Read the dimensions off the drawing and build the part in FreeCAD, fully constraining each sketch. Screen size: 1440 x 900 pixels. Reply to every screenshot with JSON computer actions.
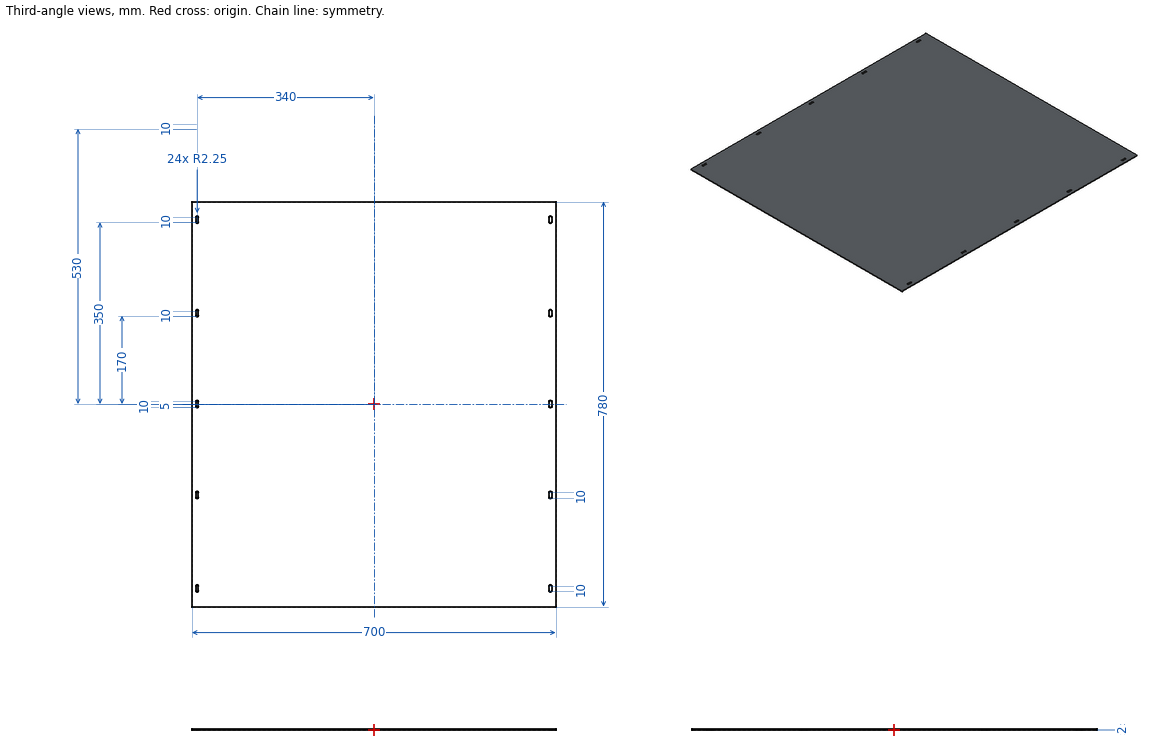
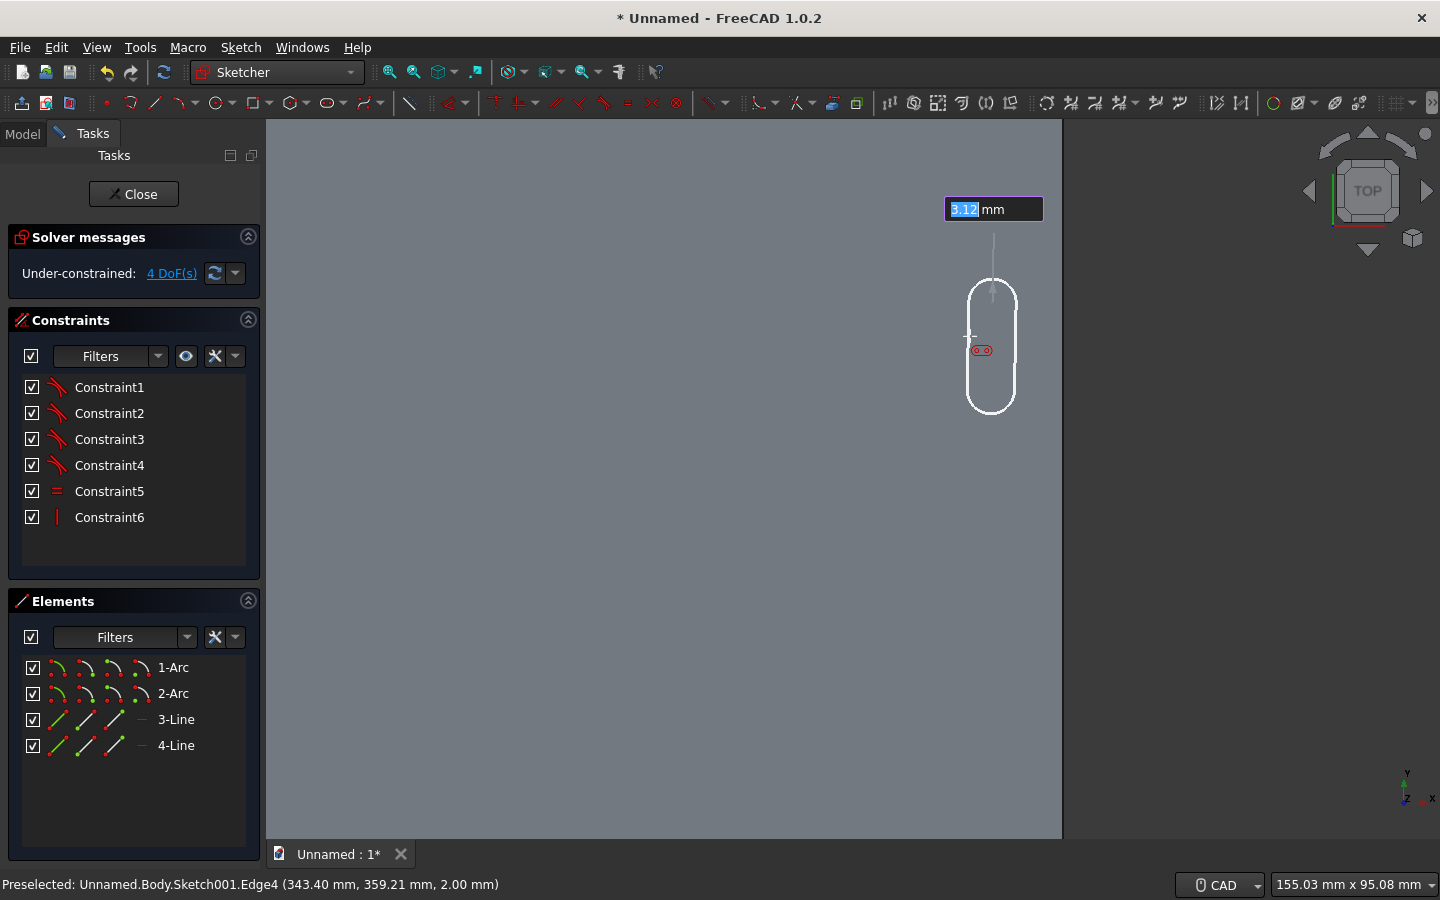
{"action": "left_click", "coordinate": [970, 335]}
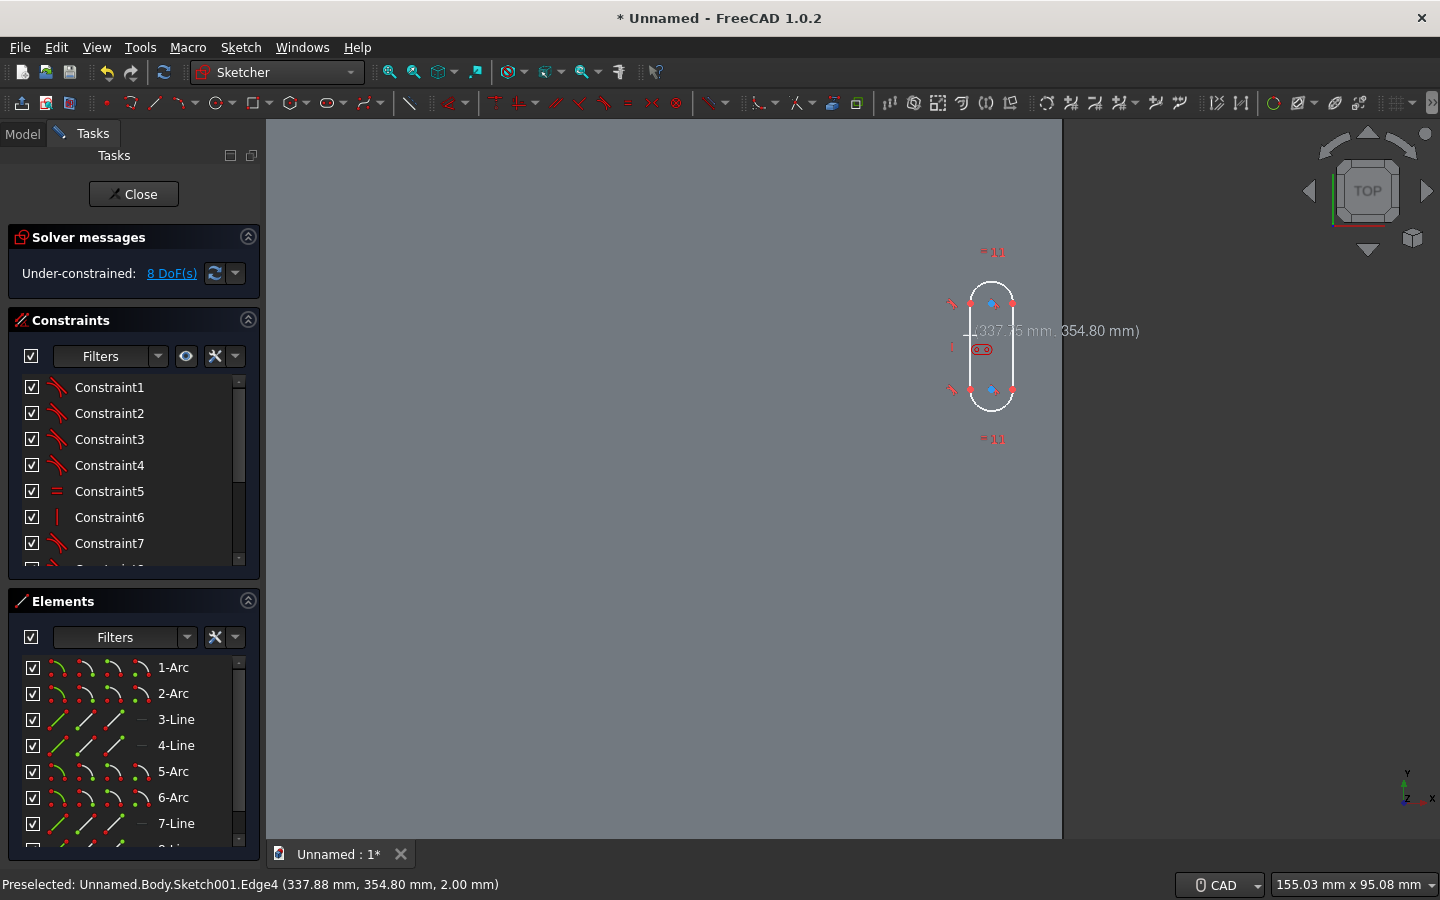
{"action": "scroll", "coordinate": [975, 330], "scroll_direction": "down", "scroll_amount": 13}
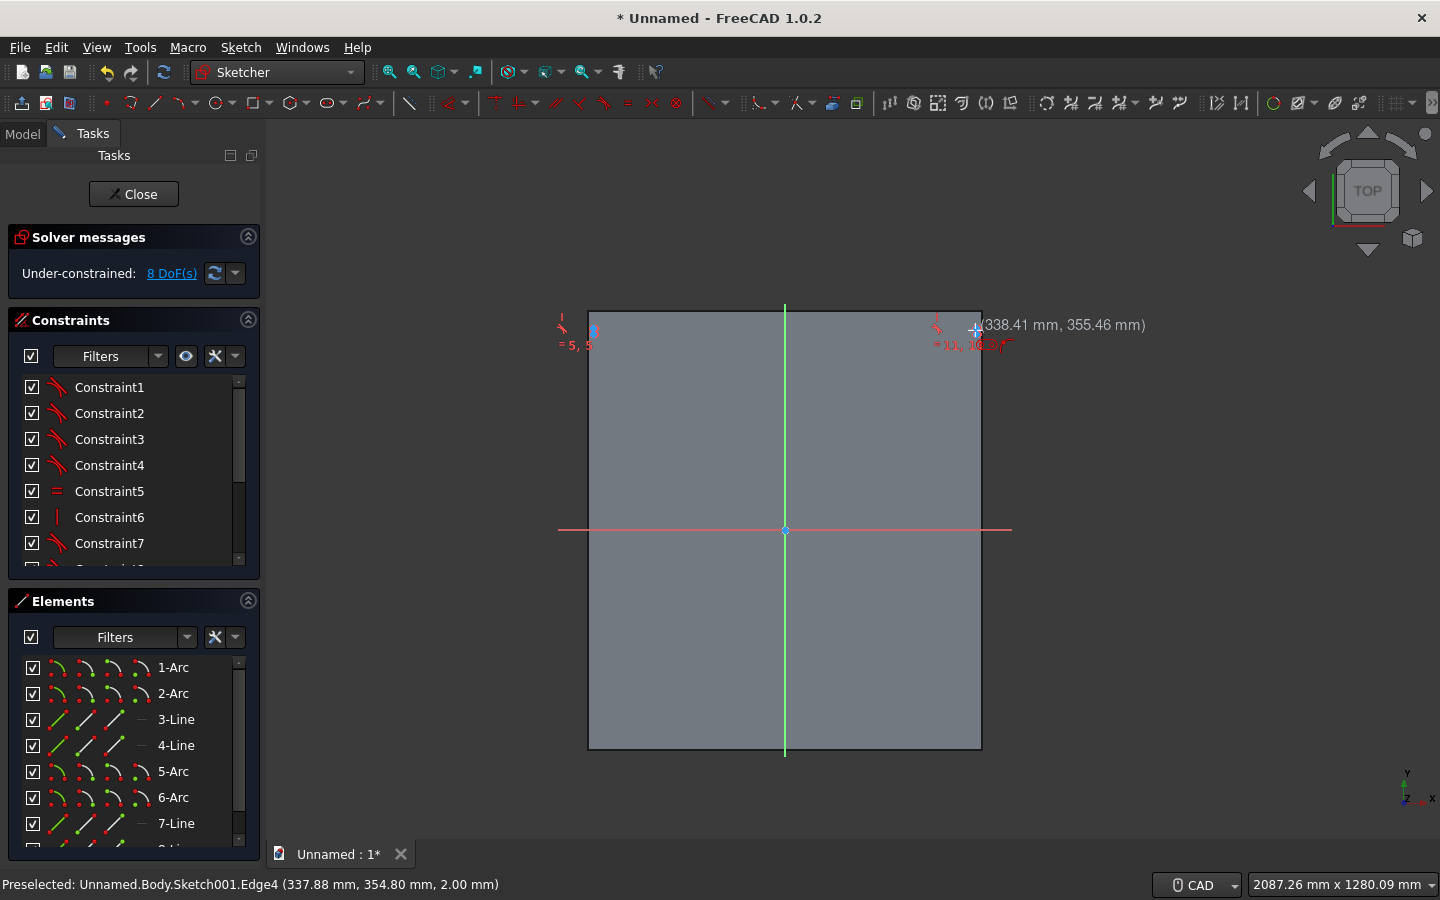
{"action": "scroll", "coordinate": [594, 435], "scroll_direction": "up", "scroll_amount": 15}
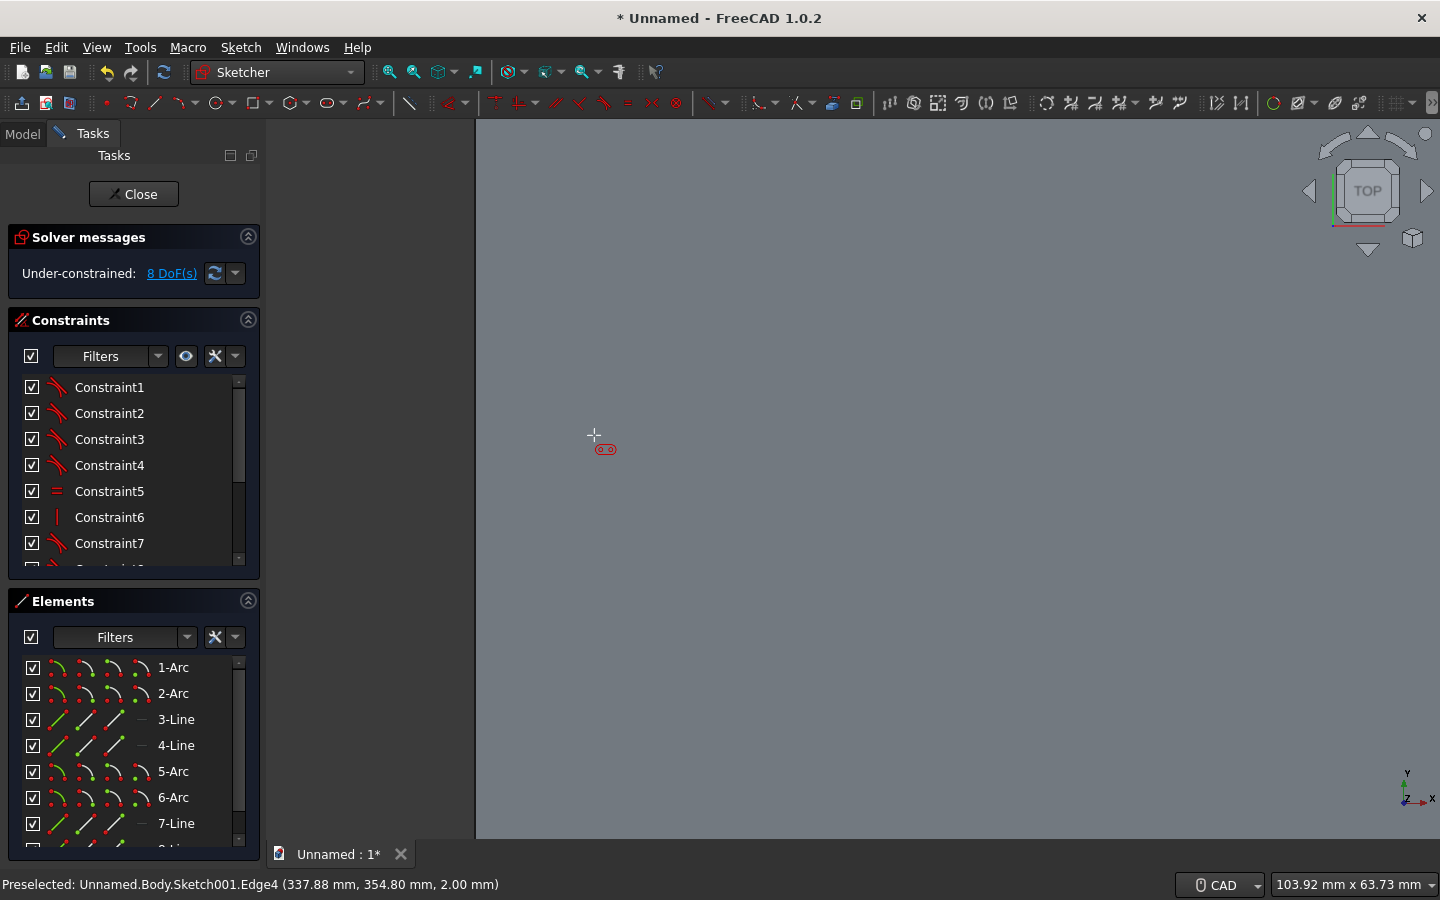
{"action": "scroll", "coordinate": [594, 435], "scroll_direction": "down", "scroll_amount": 15}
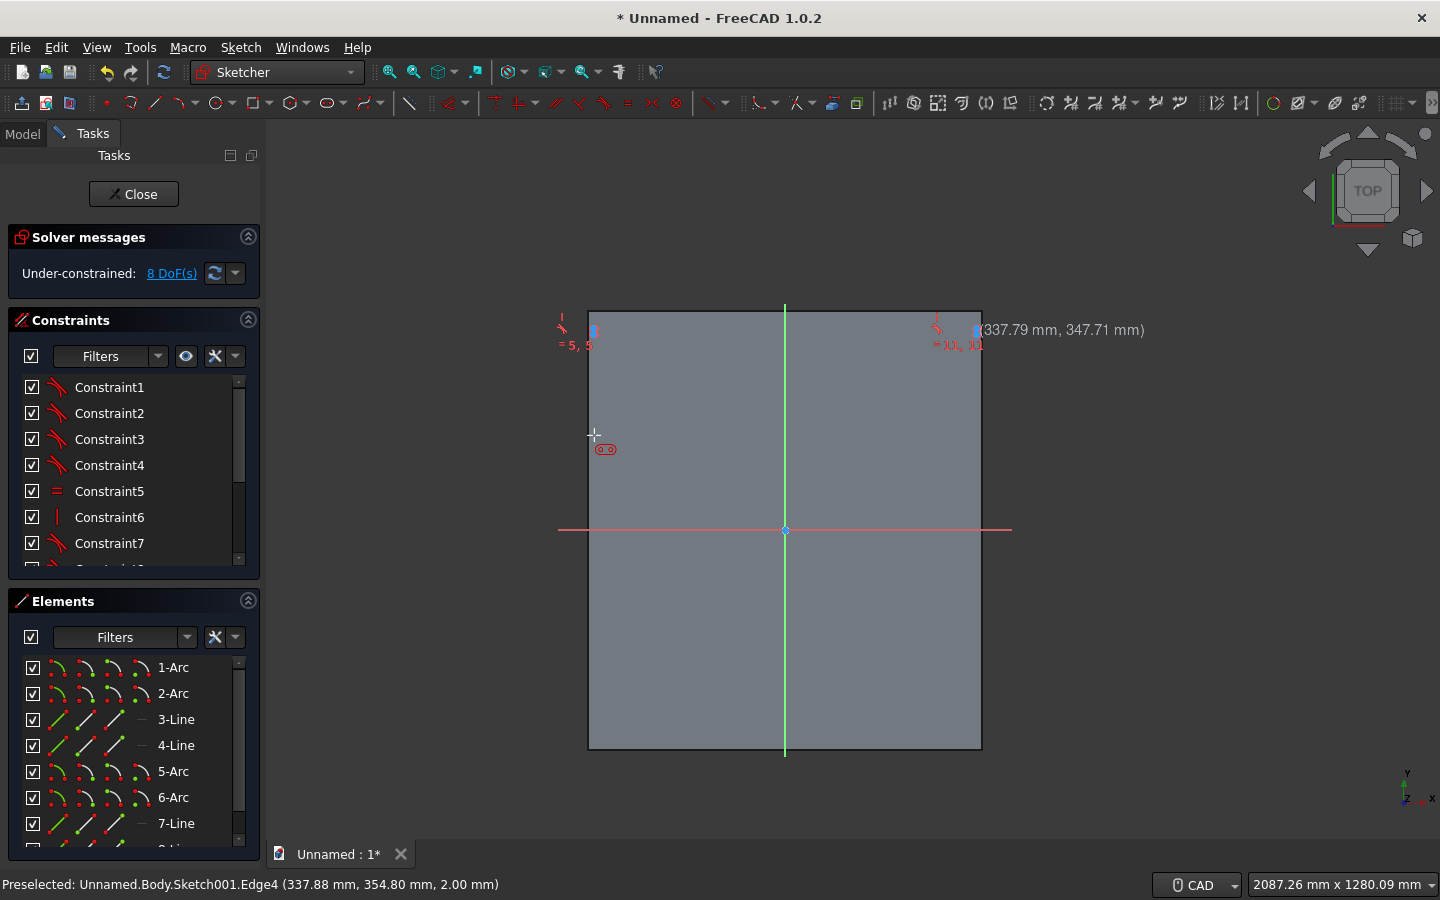
{"action": "left_click", "coordinate": [594, 435]}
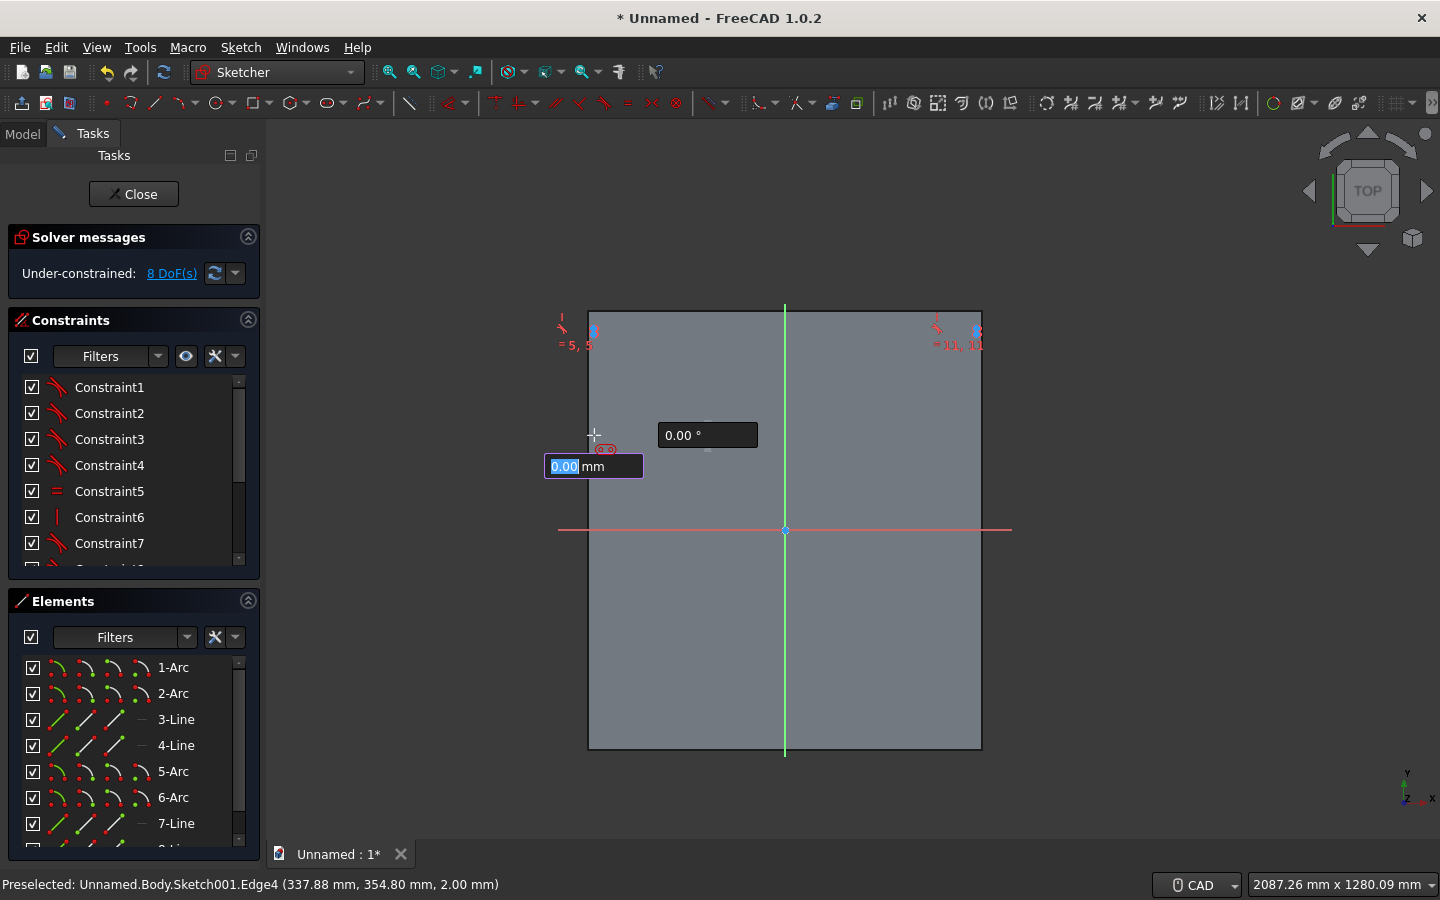
{"action": "scroll", "coordinate": [594, 429], "scroll_direction": "up", "scroll_amount": 6}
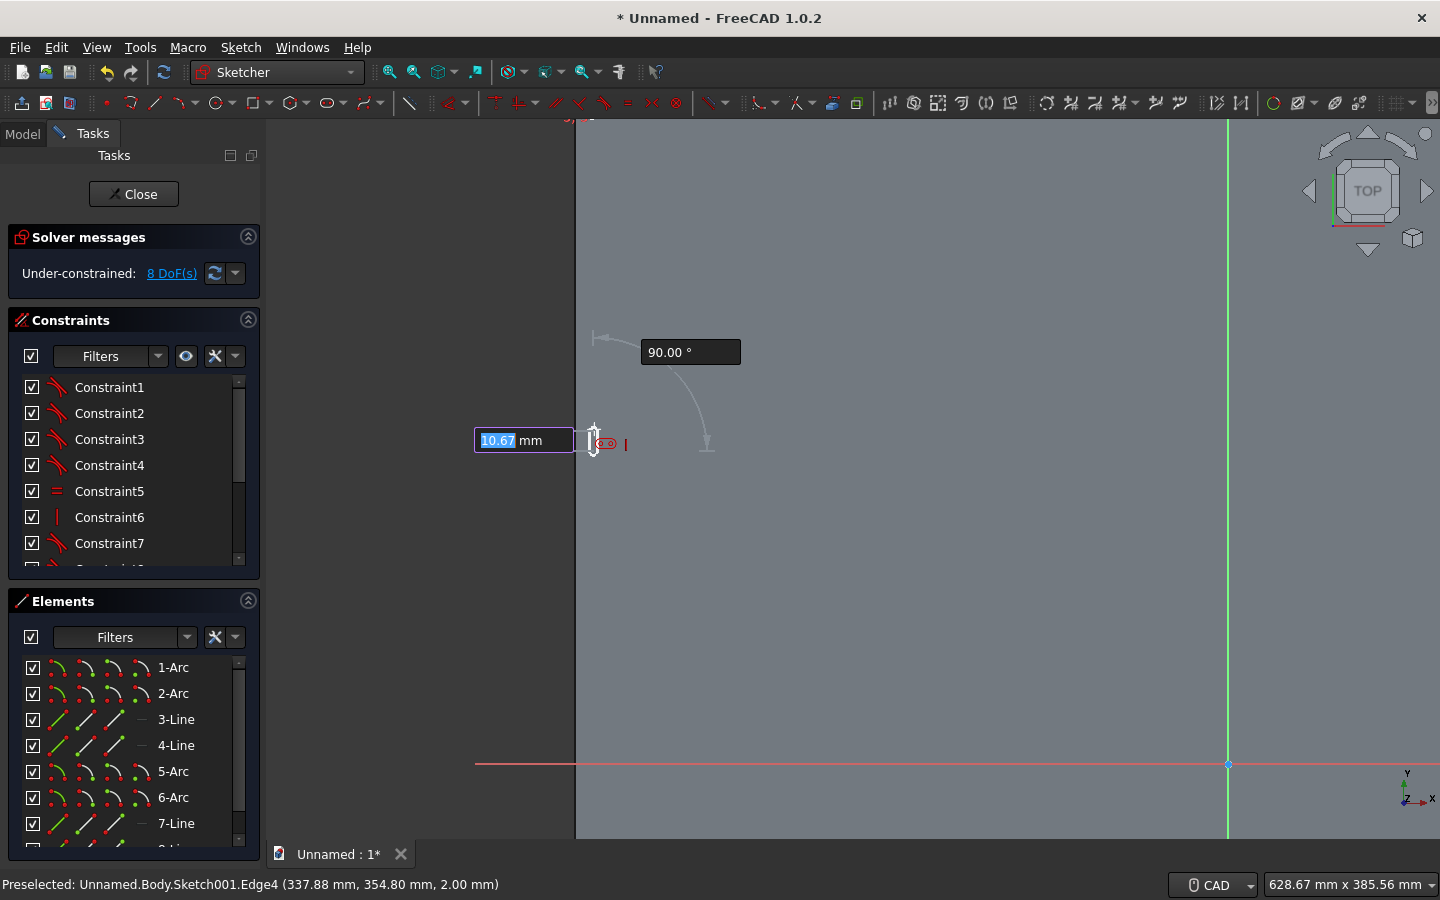
{"action": "left_click", "coordinate": [593, 428]}